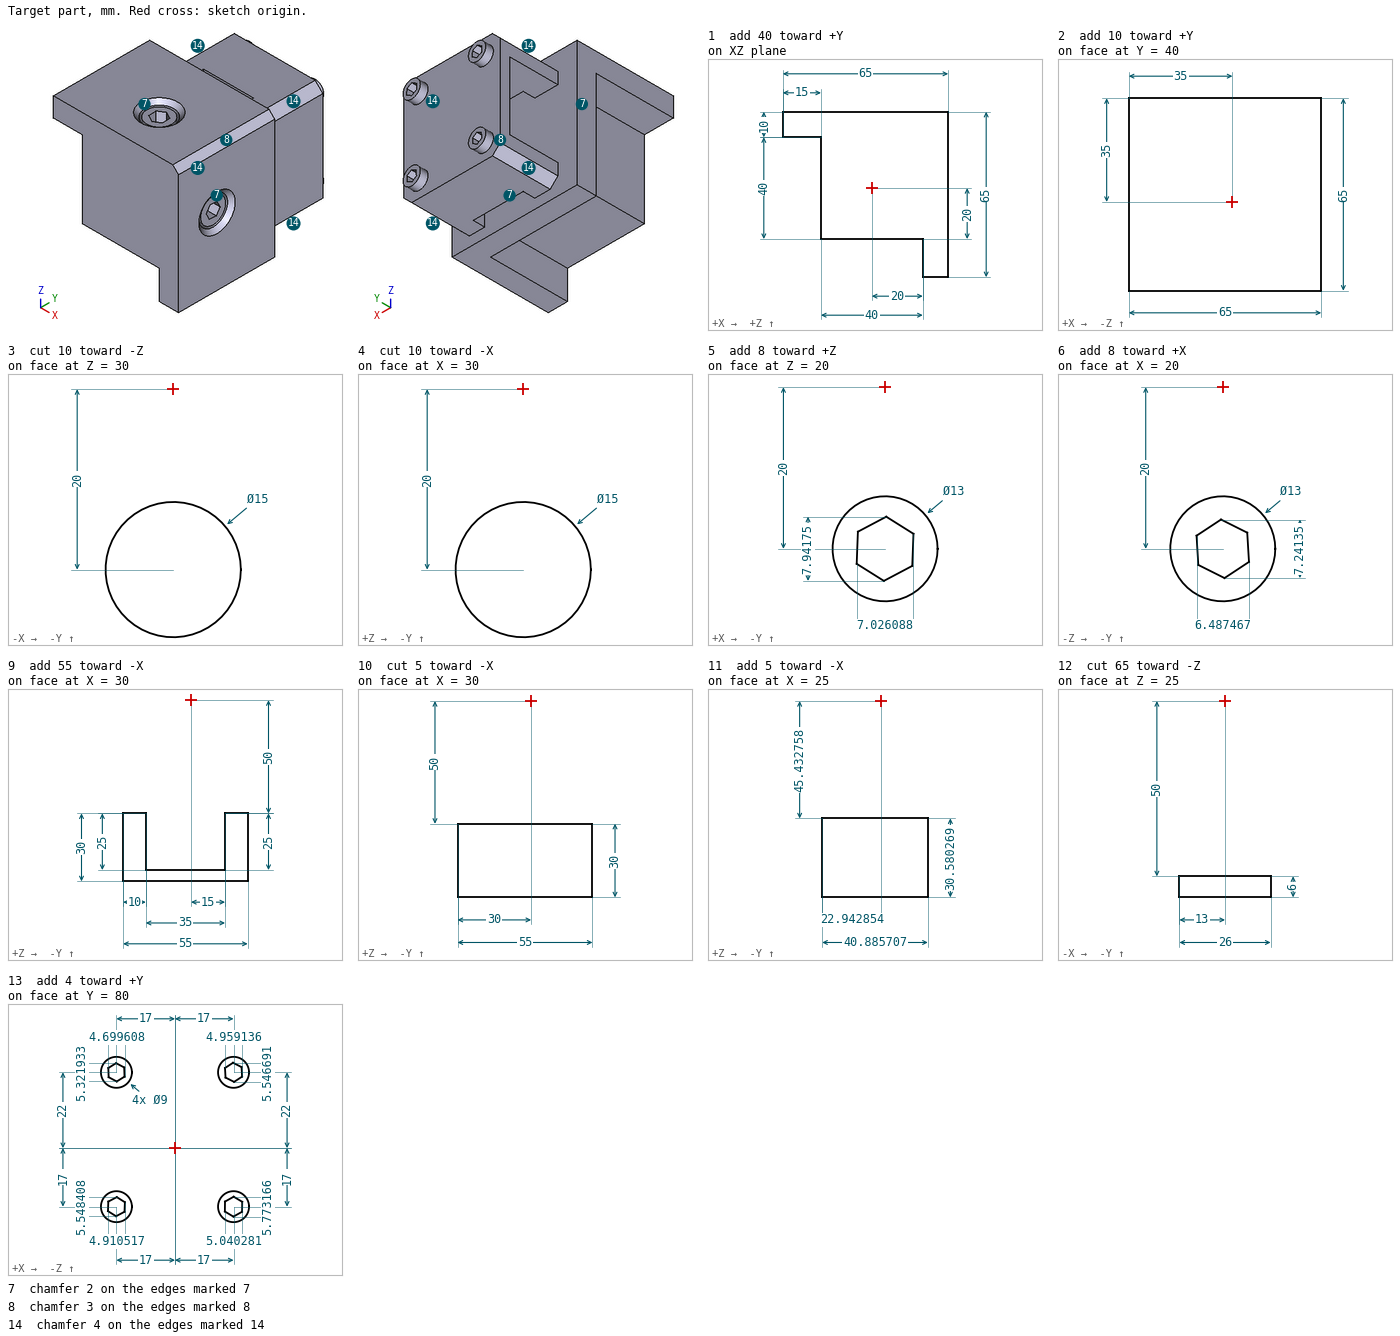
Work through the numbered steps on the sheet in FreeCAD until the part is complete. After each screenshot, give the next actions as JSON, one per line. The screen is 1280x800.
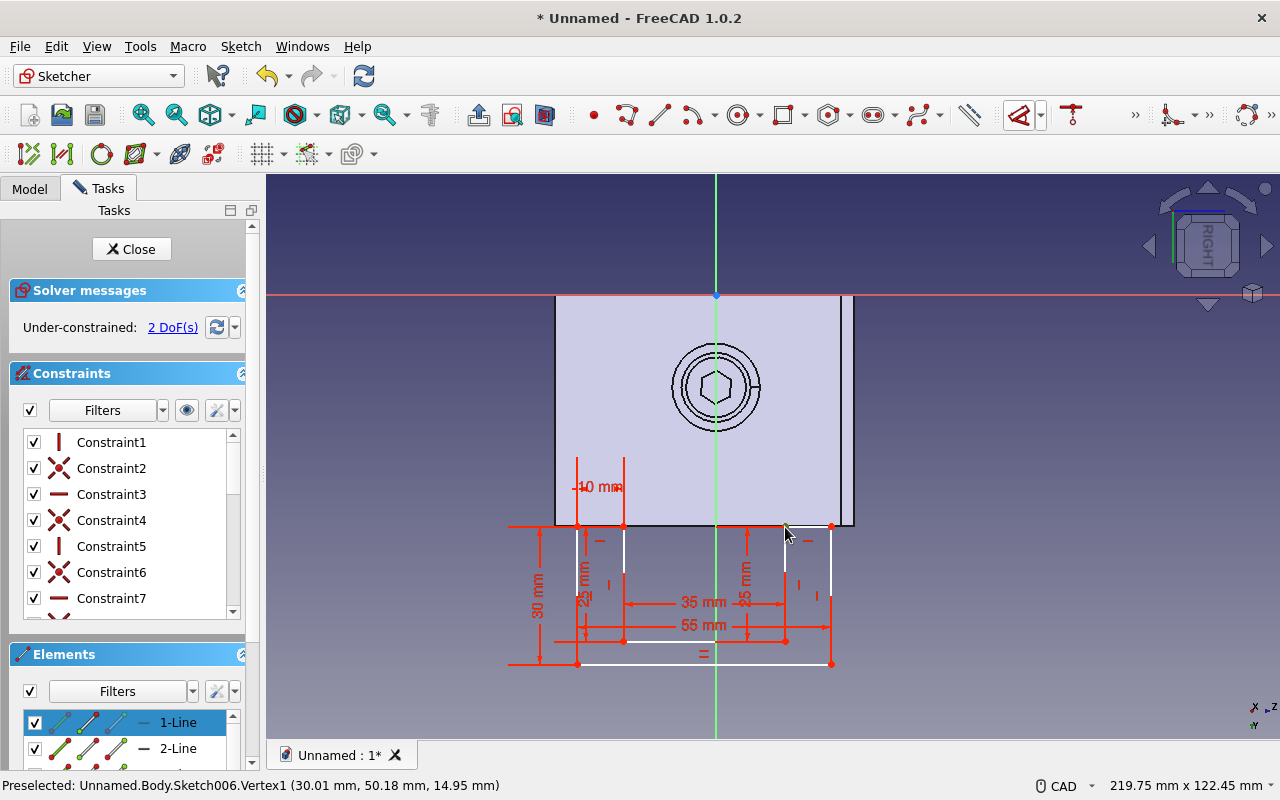
{"action": "key", "text": "l"}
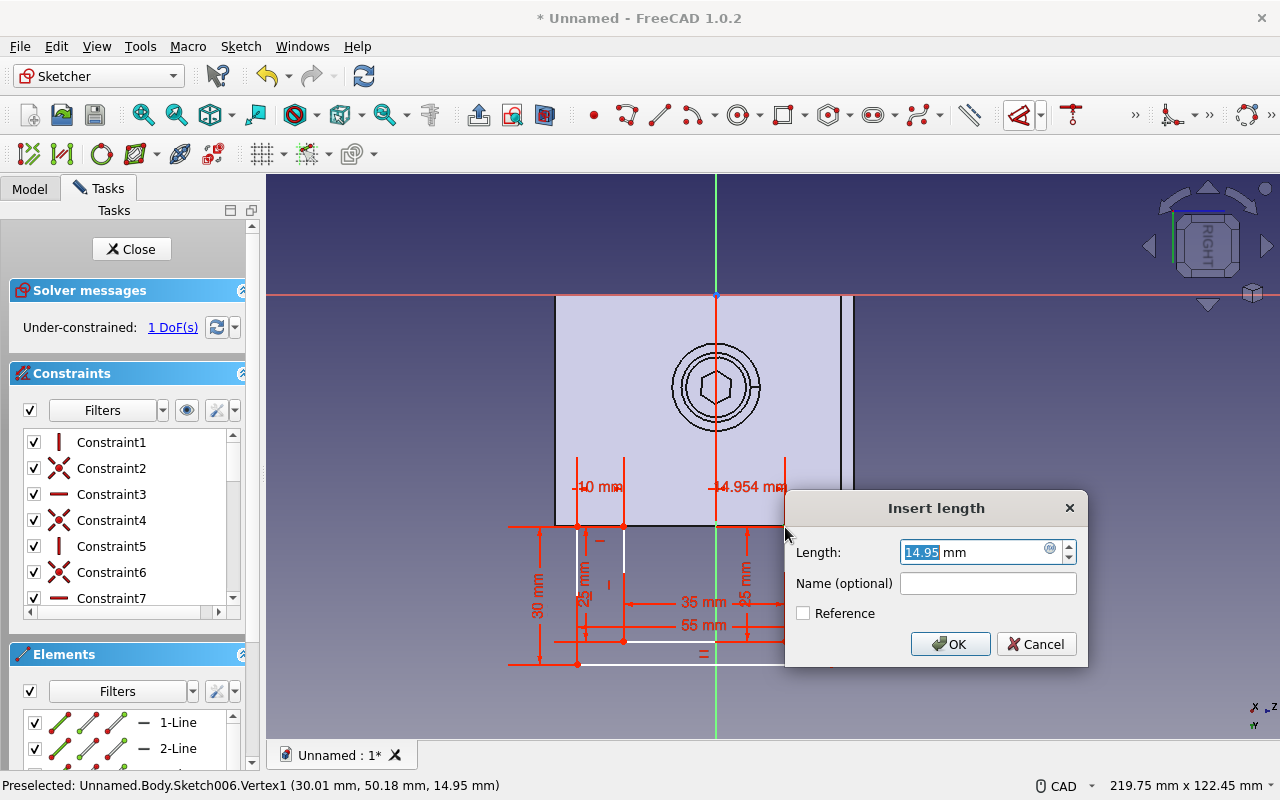
{"action": "type", "text": "15"}
{"action": "key", "text": "Return"}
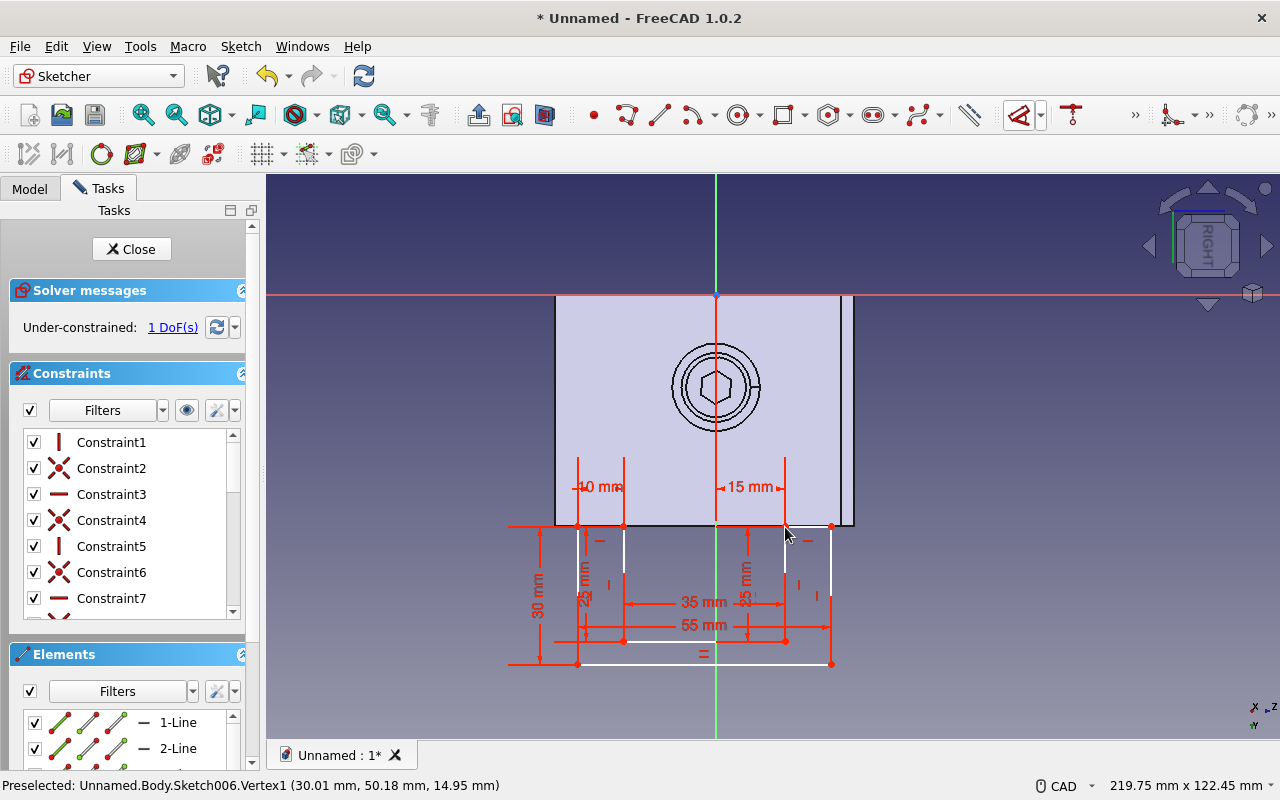
{"action": "left_click", "coordinate": [785, 527]}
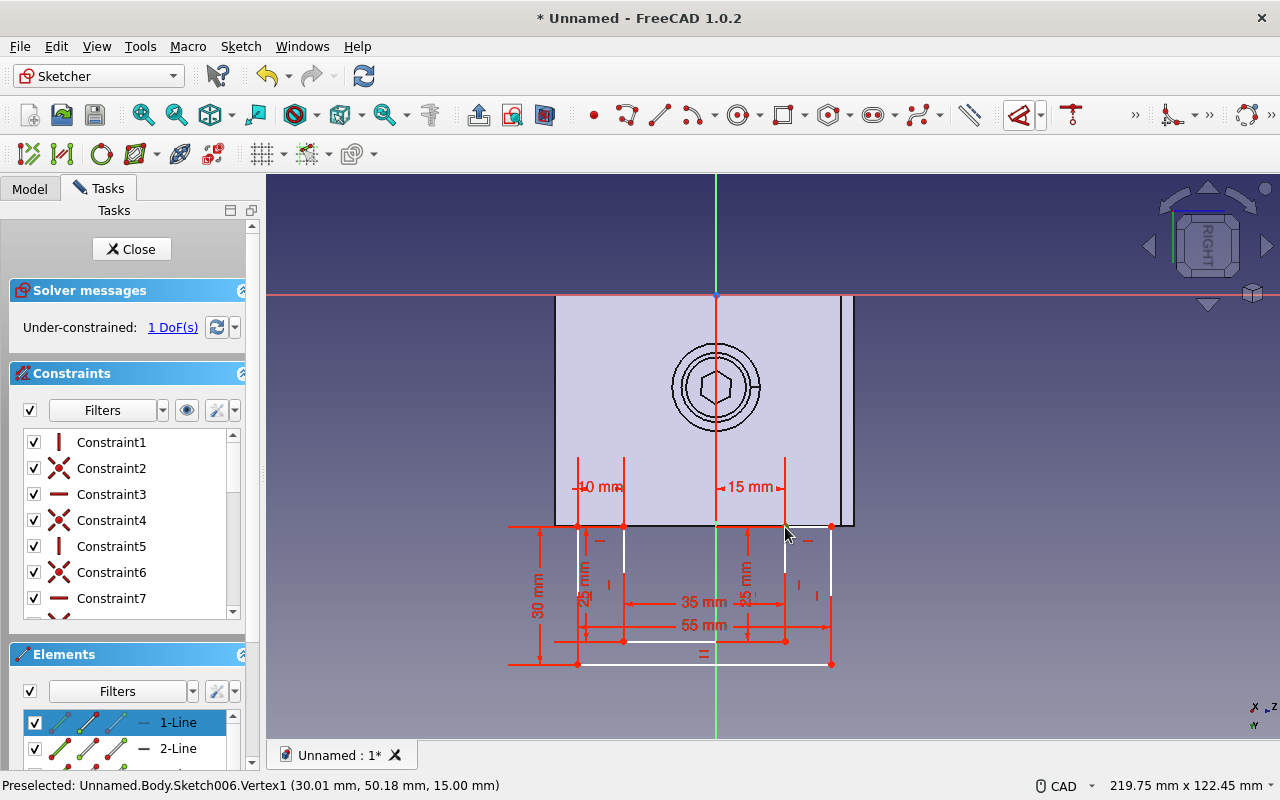
{"action": "key", "text": "i"}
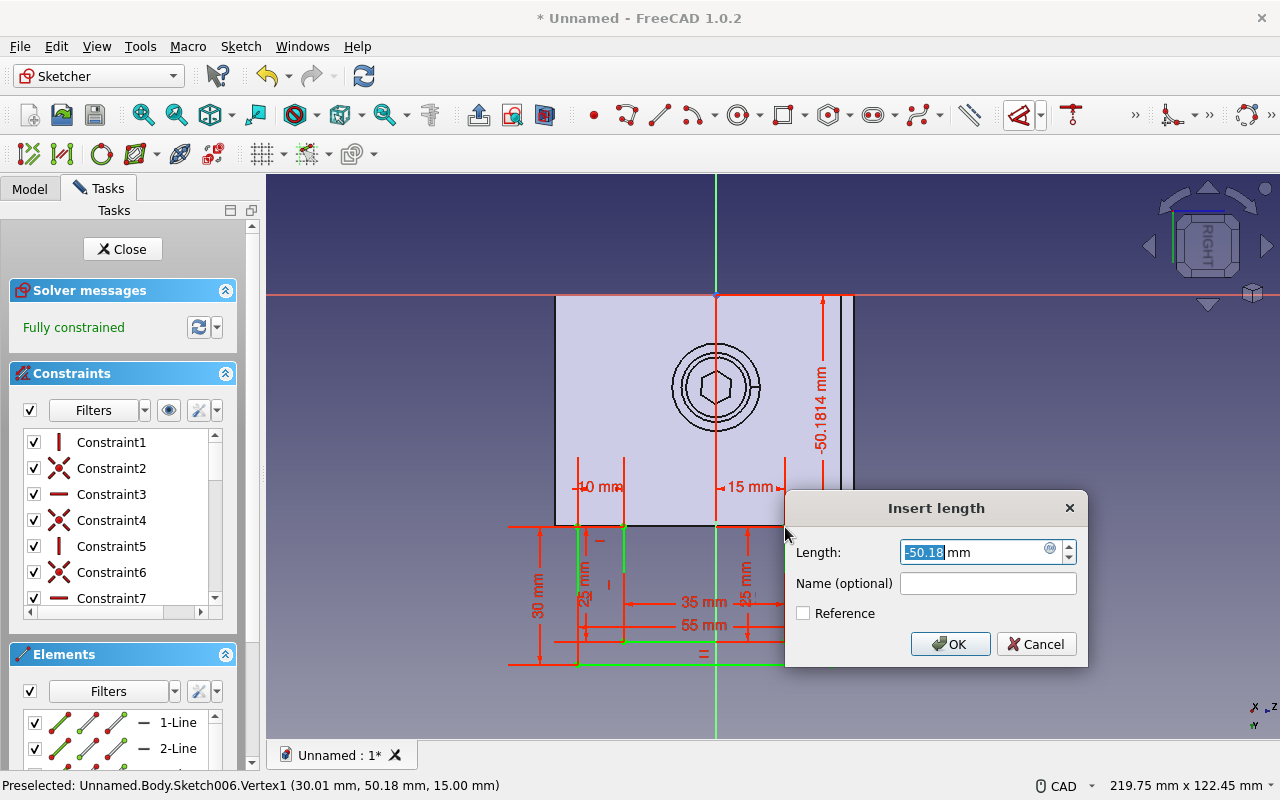
{"action": "type", "text": "-50"}
{"action": "key", "text": "Return"}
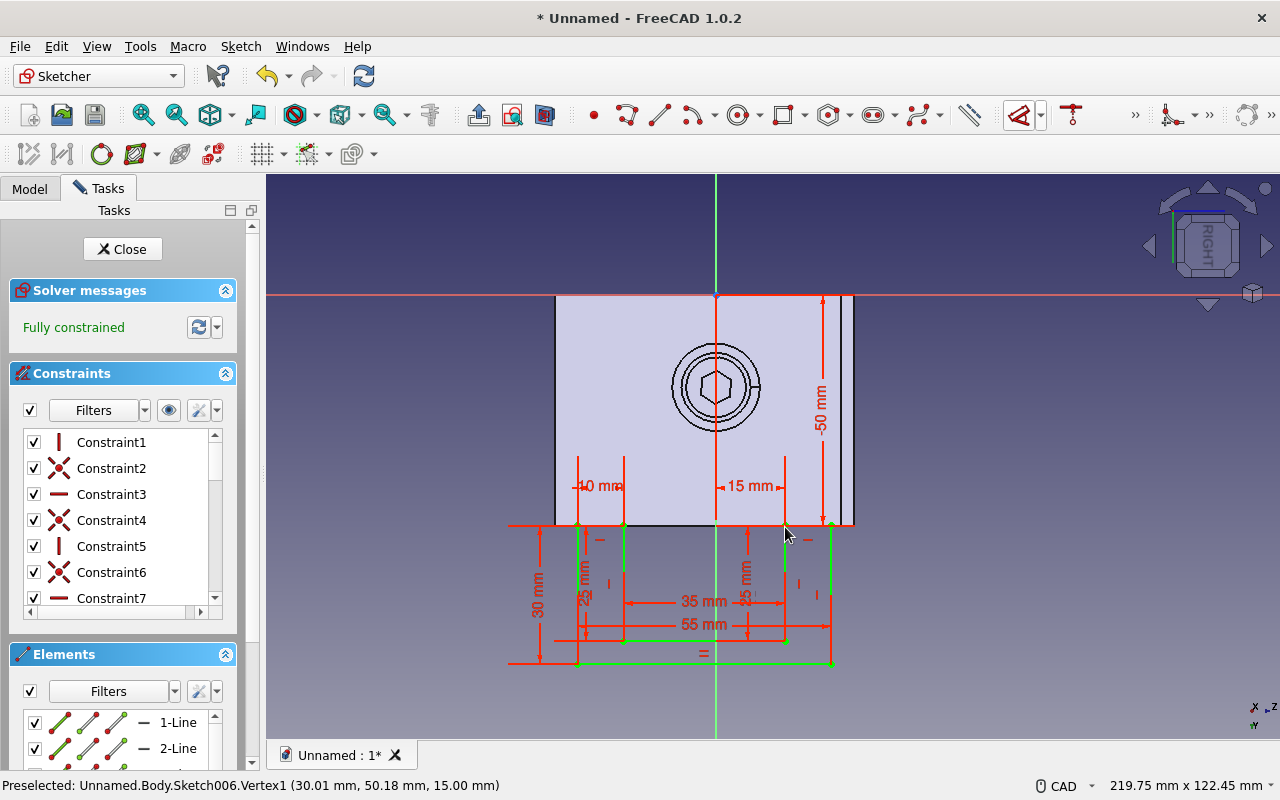
{"action": "left_click", "coordinate": [123, 249]}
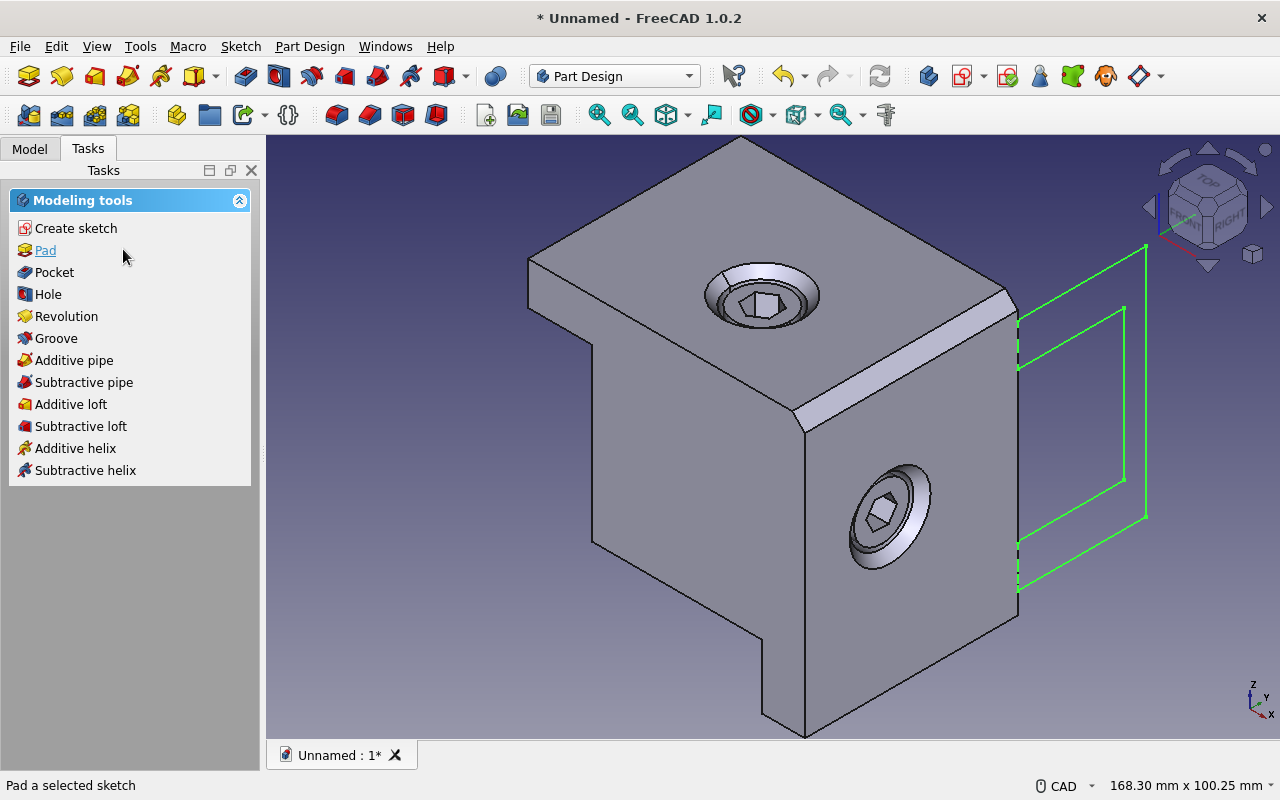
{"action": "left_click", "coordinate": [29, 76]}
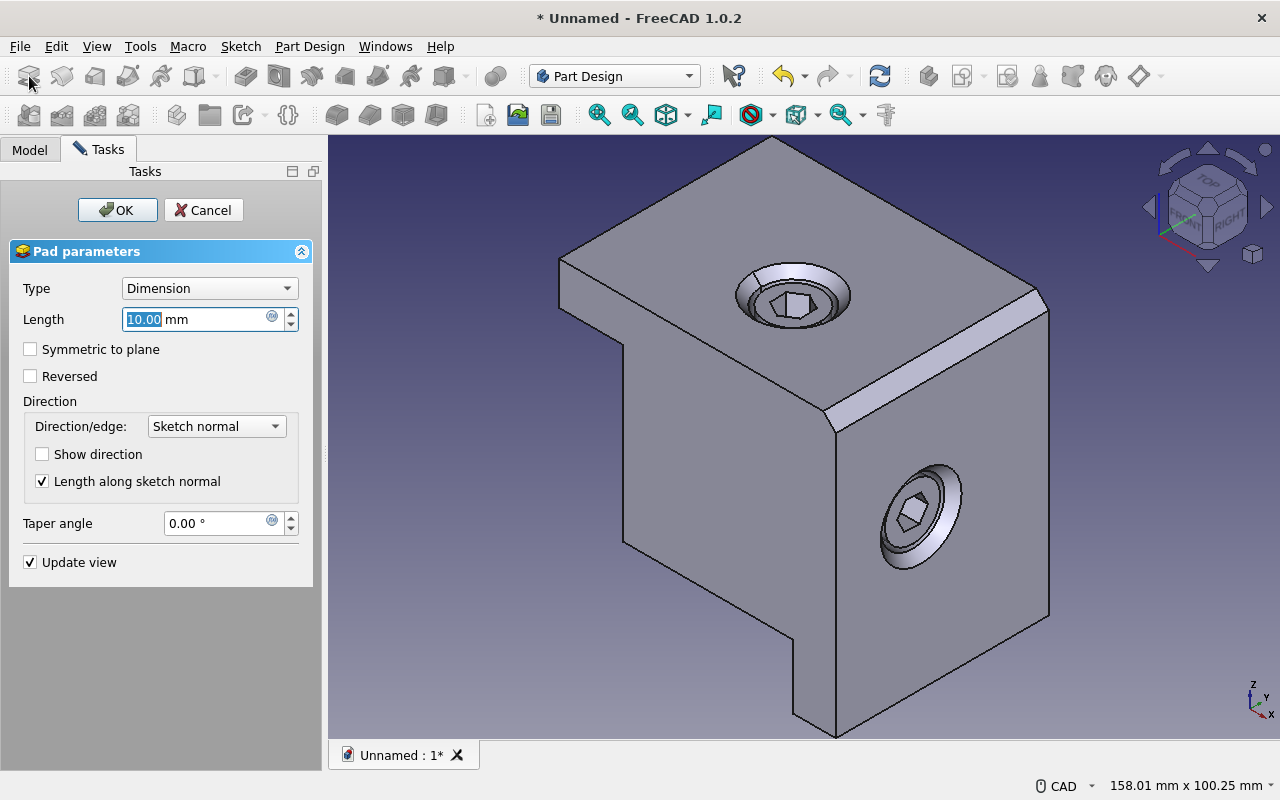
{"action": "type", "text": "55"}
{"action": "key", "text": "Tab"}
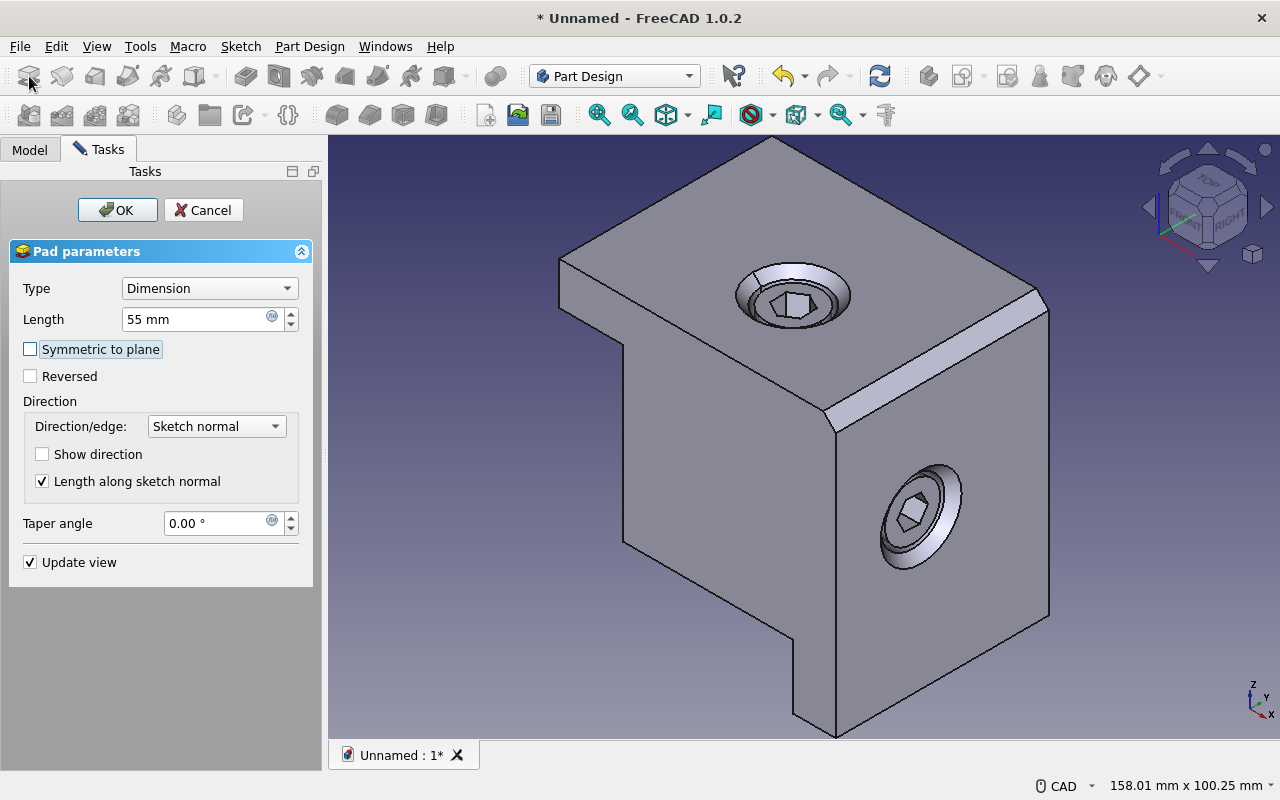
{"action": "left_click", "coordinate": [31, 376]}